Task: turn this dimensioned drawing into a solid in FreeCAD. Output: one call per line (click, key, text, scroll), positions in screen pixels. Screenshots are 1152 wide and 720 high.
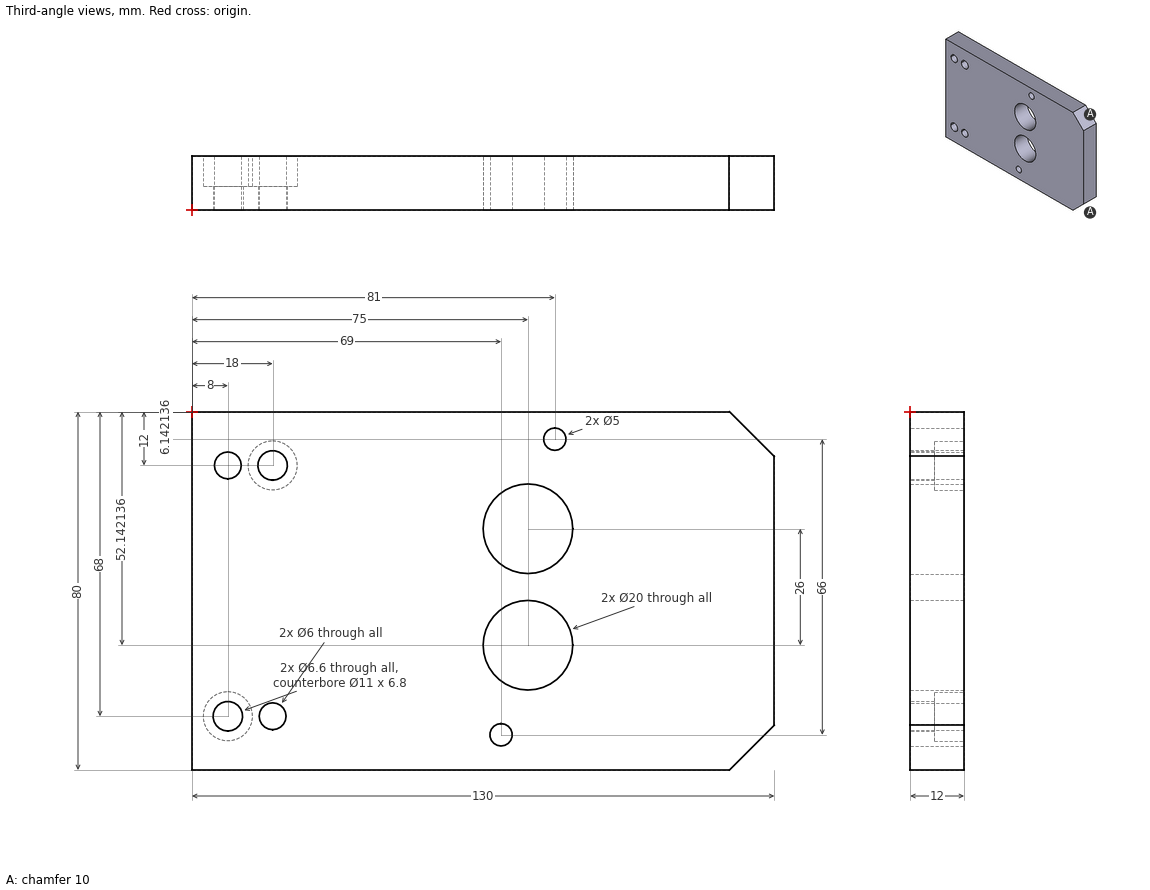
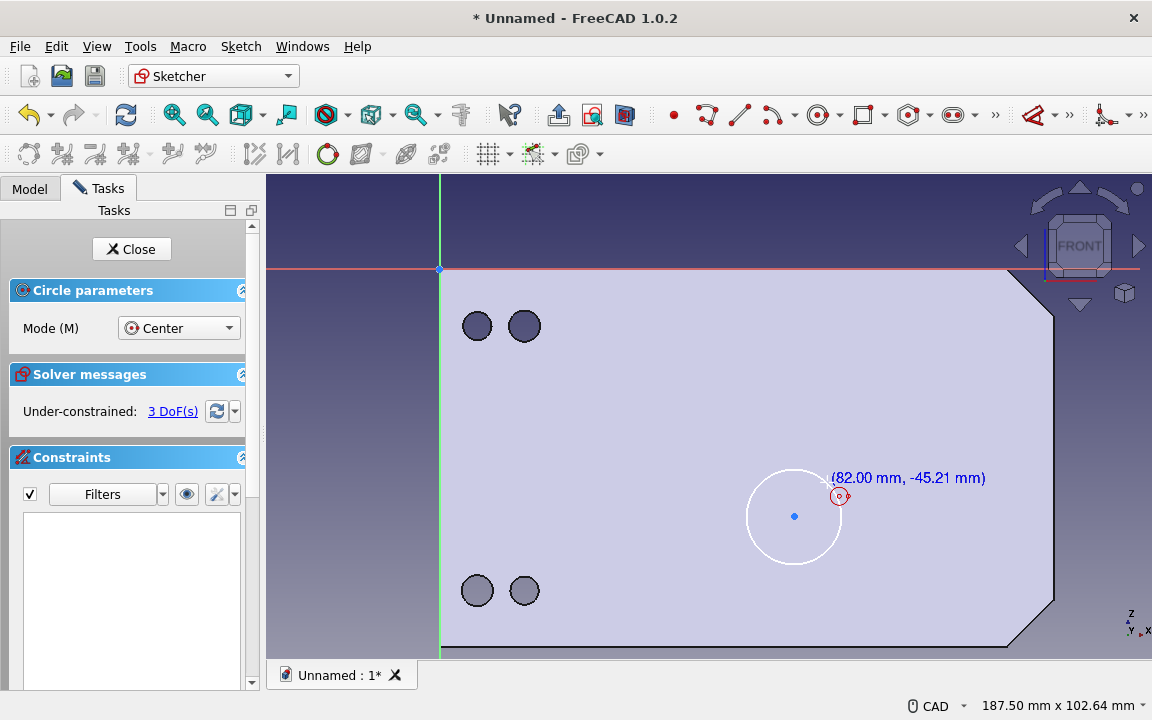
click(794, 393)
click(827, 359)
key(Escape)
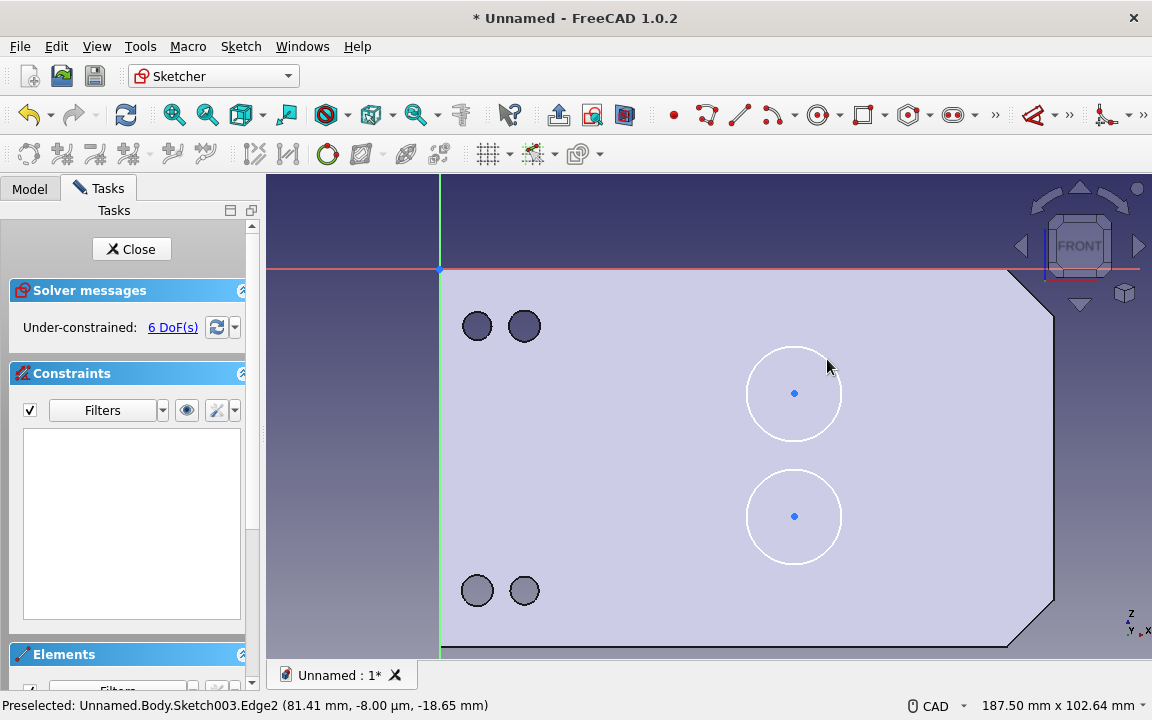
click(827, 483)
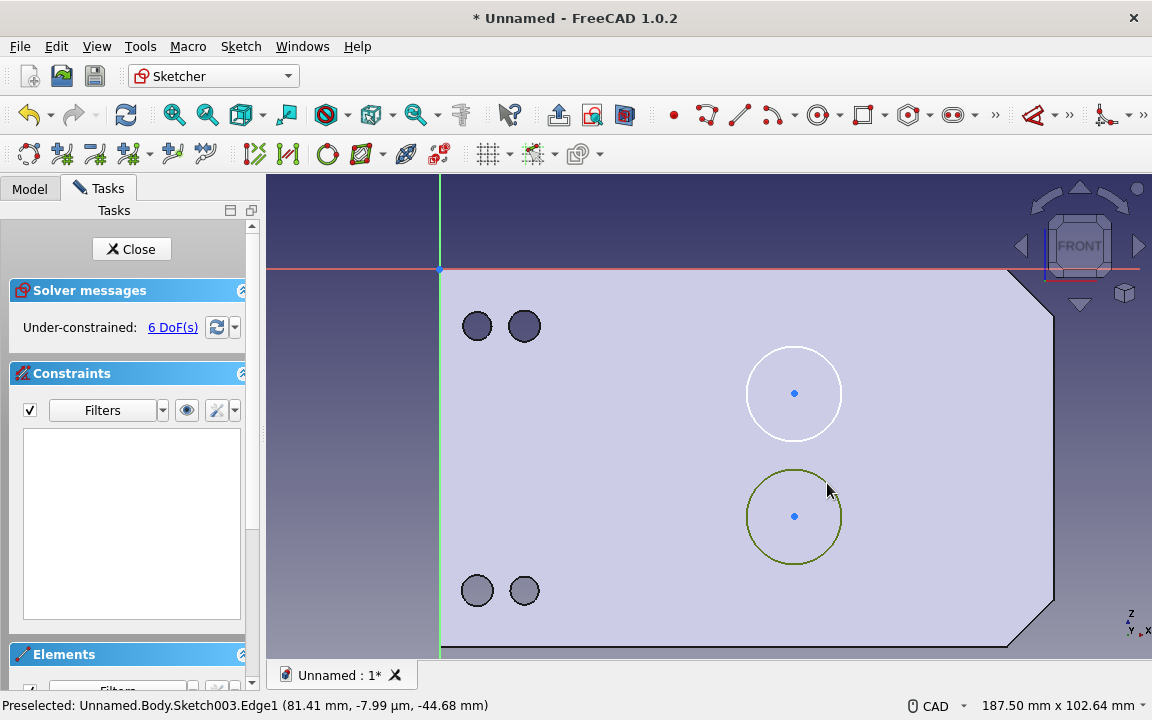
click(827, 360)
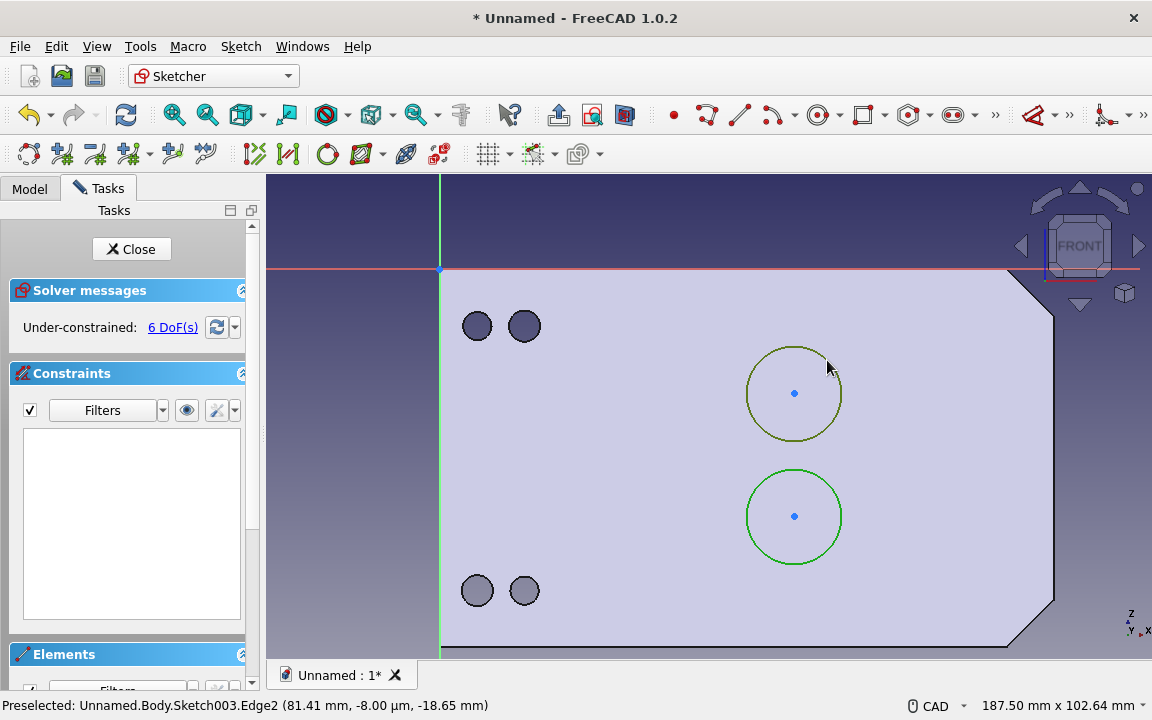
key(e)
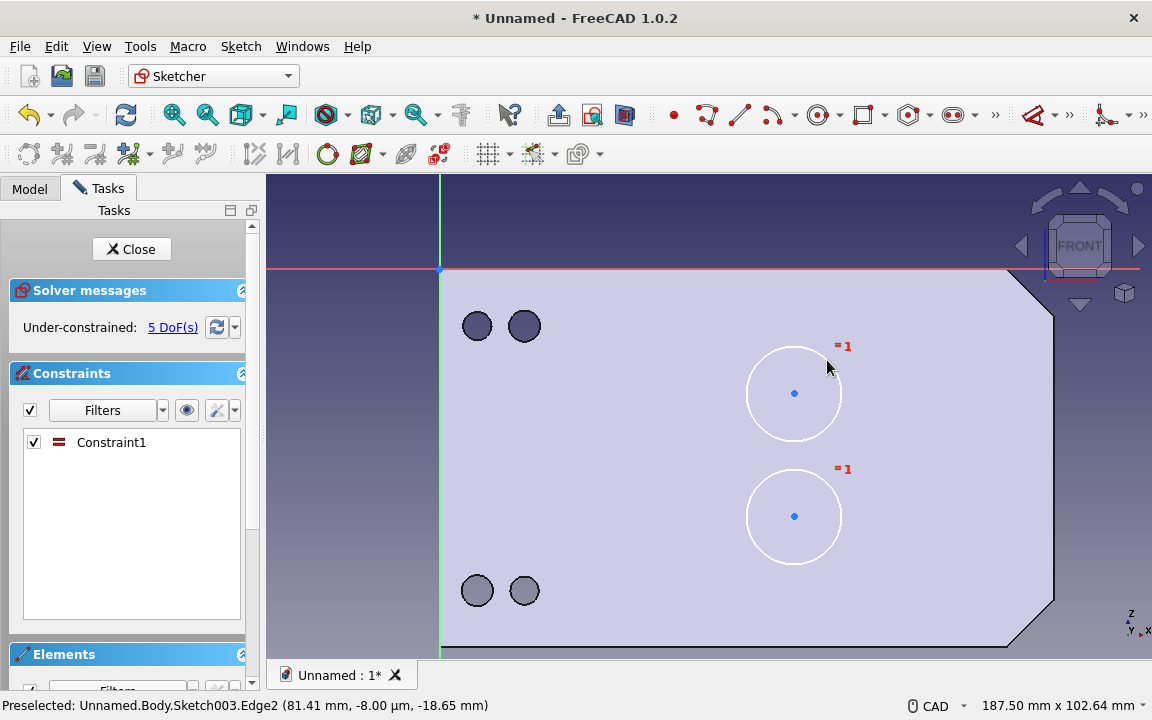
key(d)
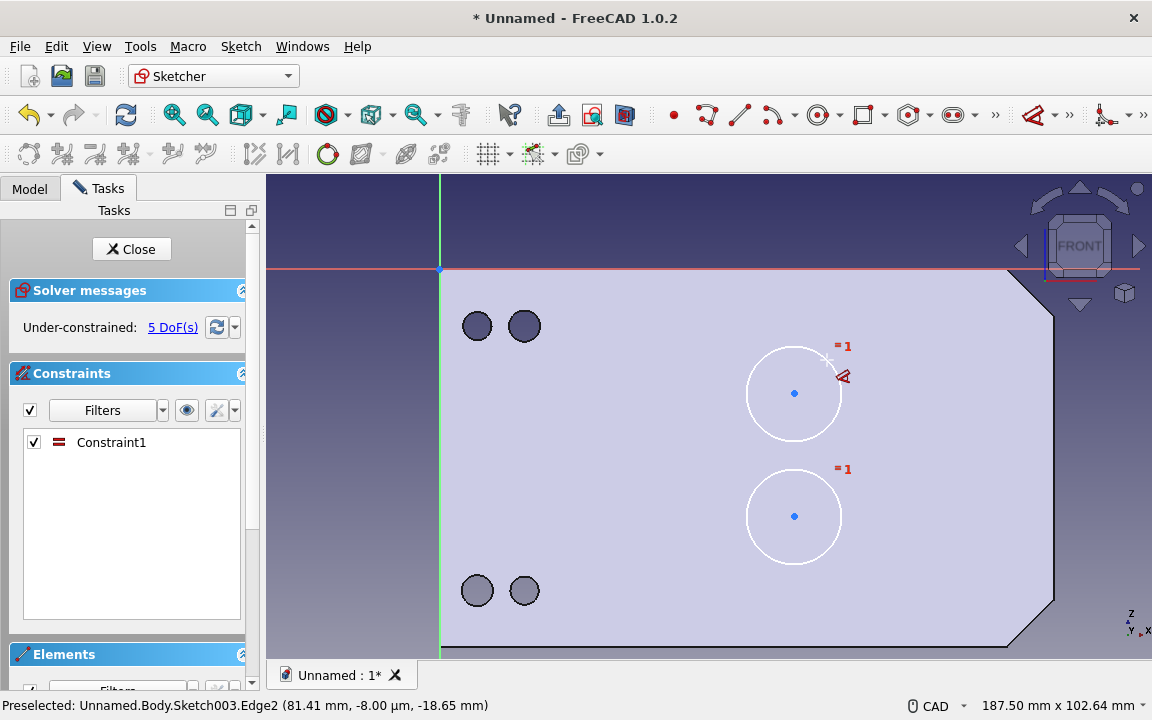
click(827, 483)
click(849, 460)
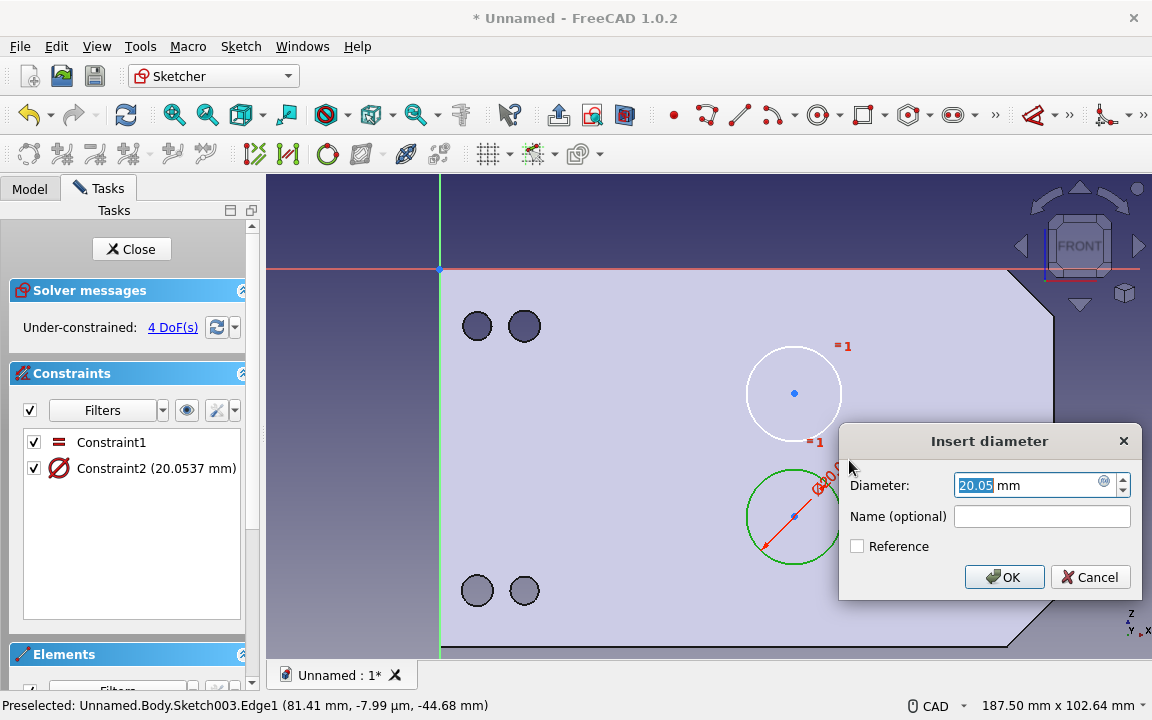
text(20)
key(Return)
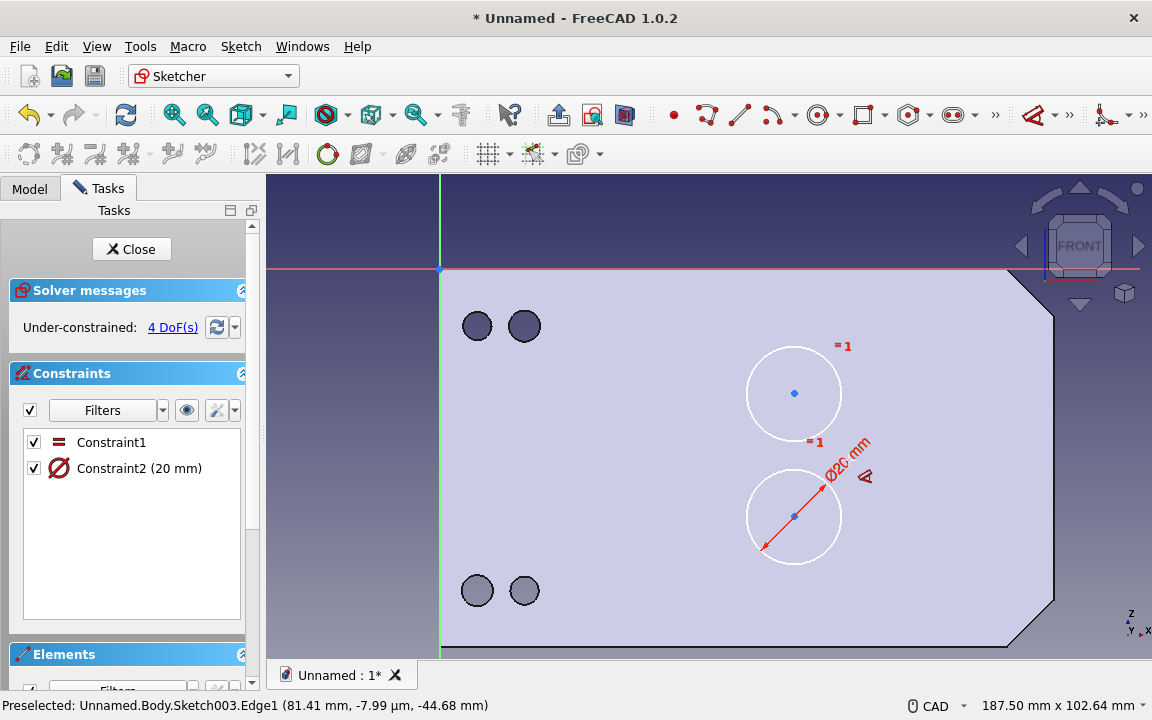
click(794, 517)
click(617, 235)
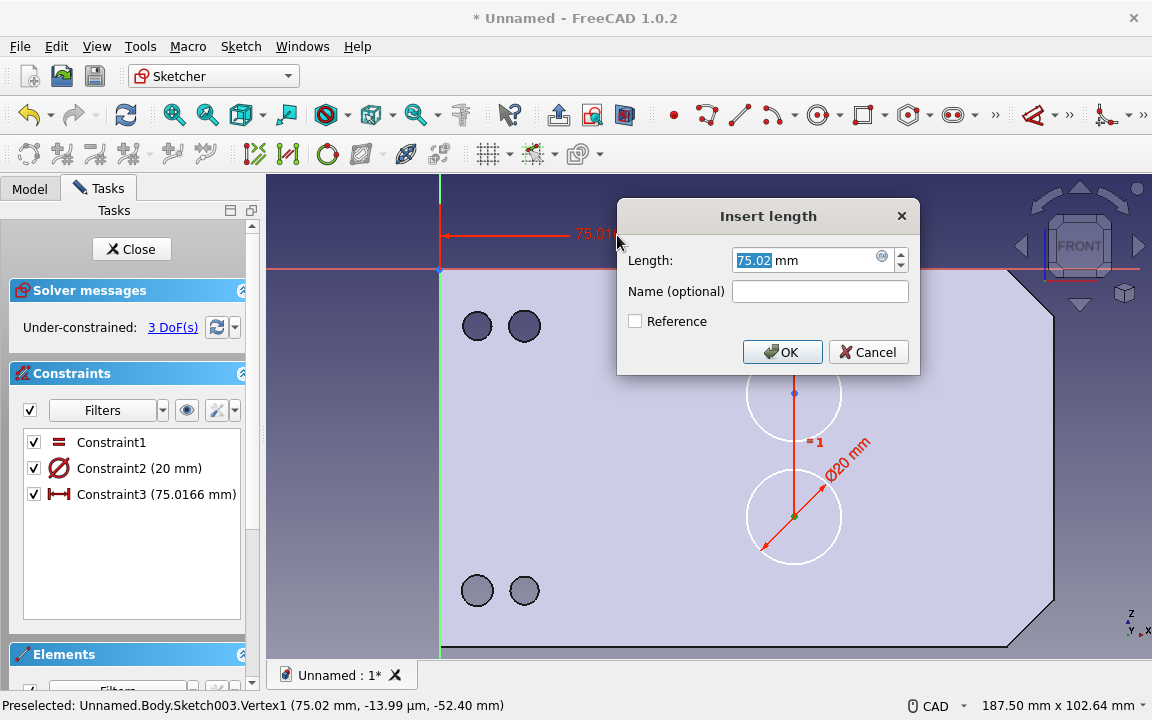
text(75)
key(Return)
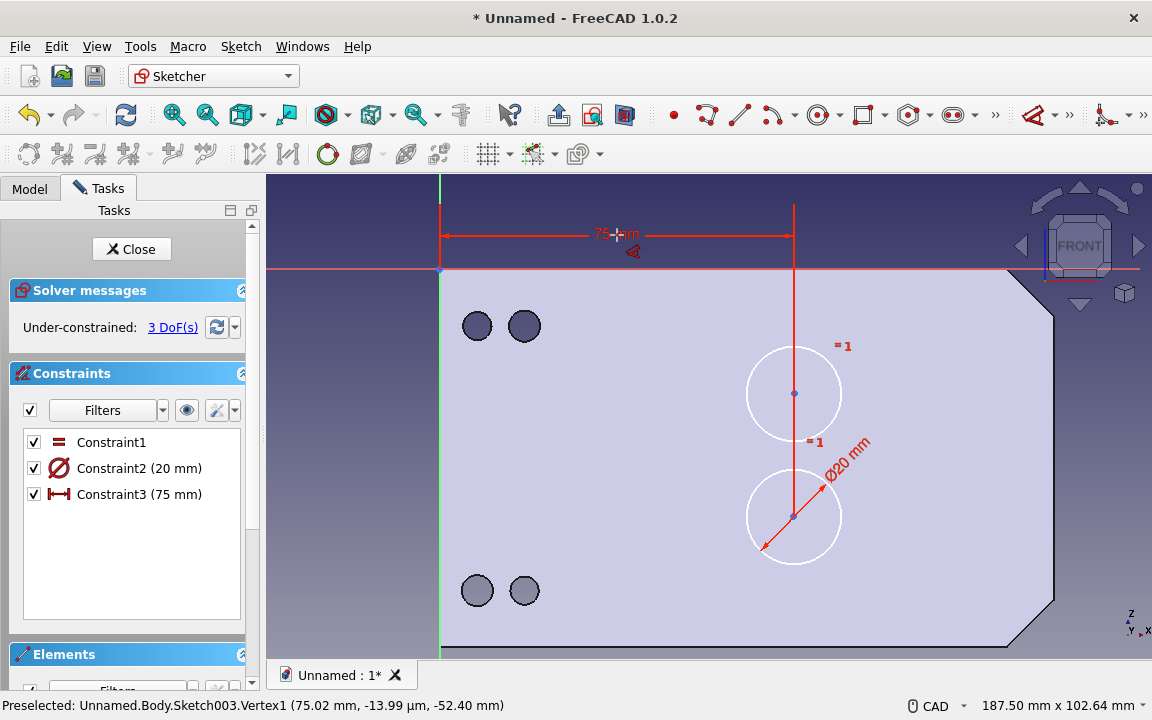
click(794, 394)
click(535, 235)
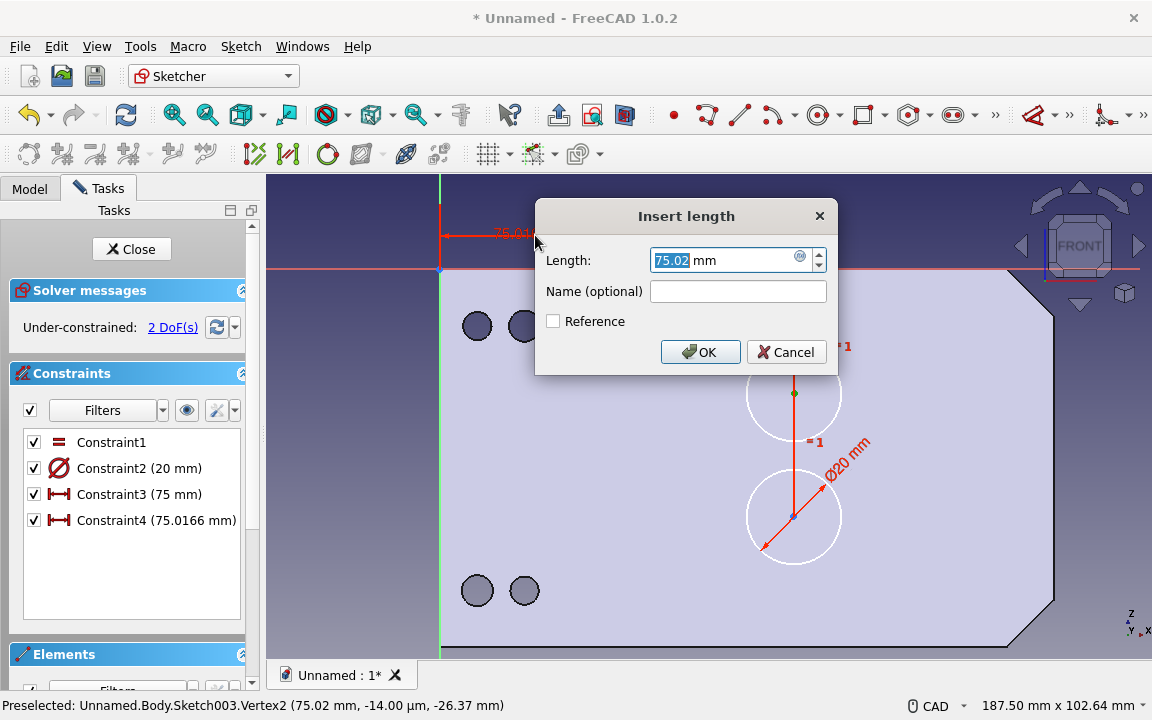
text(75)
key(Return)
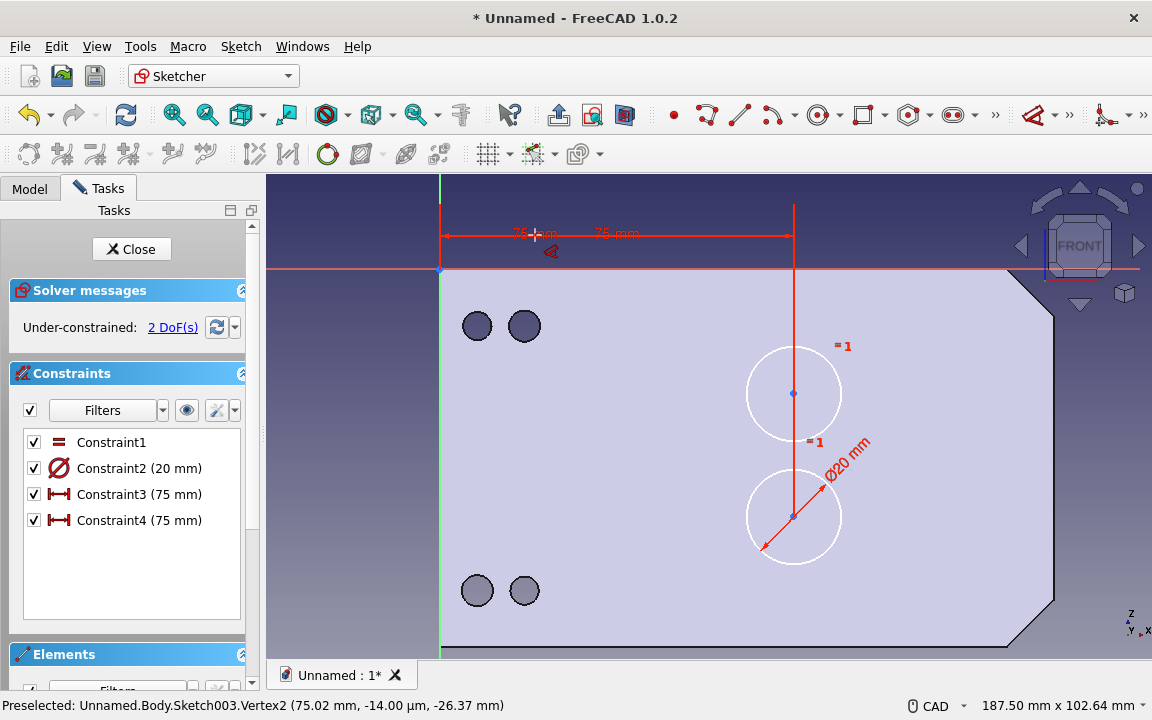
click(794, 517)